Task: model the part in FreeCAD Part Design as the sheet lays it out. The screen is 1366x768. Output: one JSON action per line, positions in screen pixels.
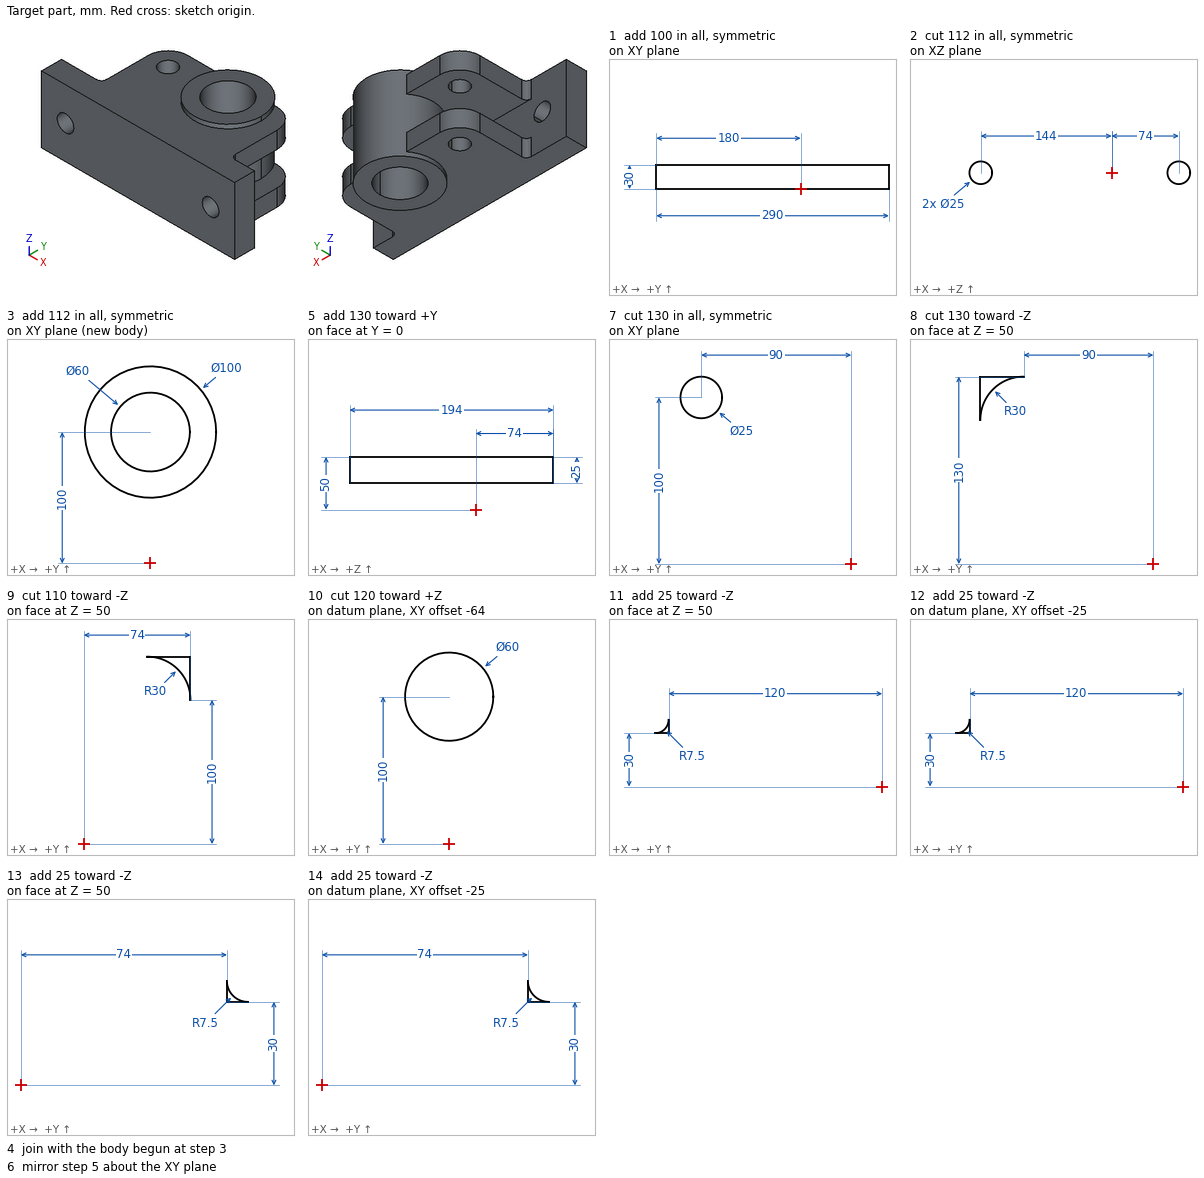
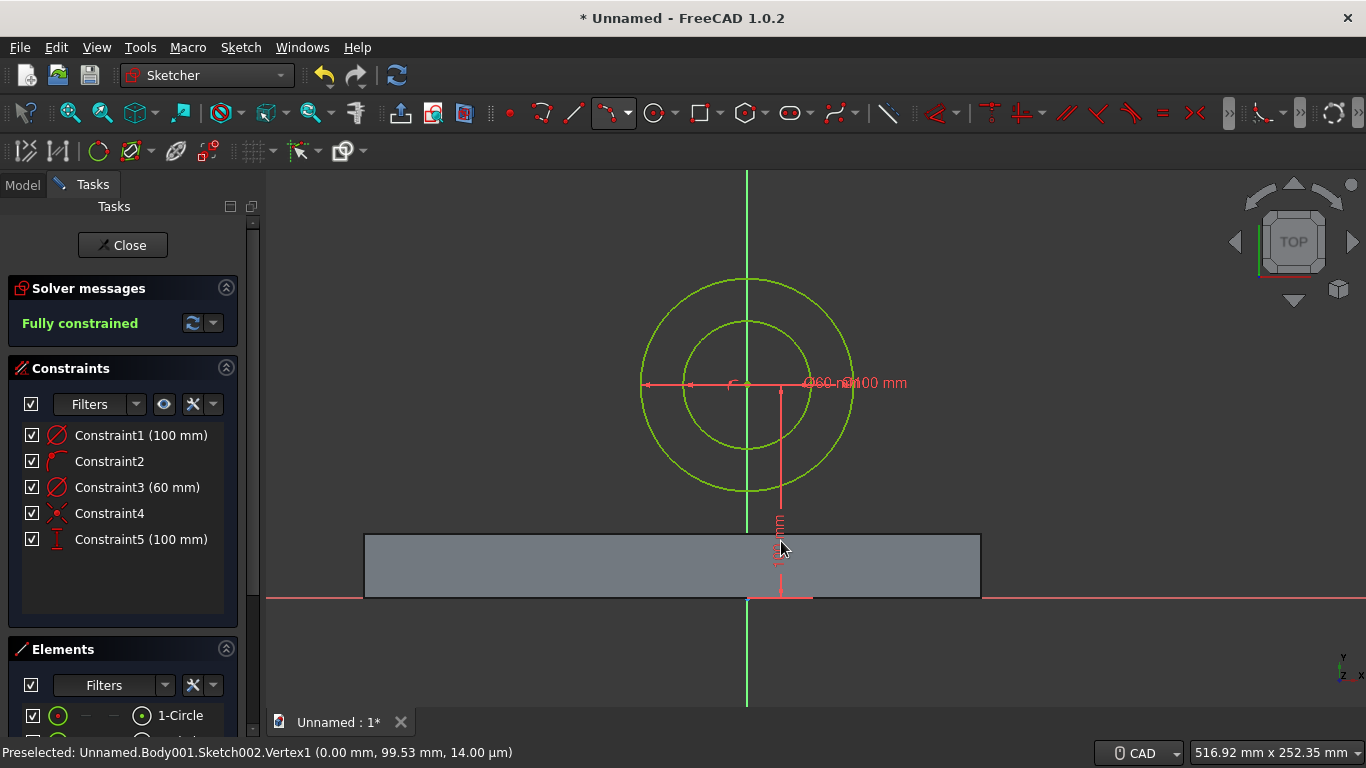
{"action": "left_click", "coordinate": [123, 245]}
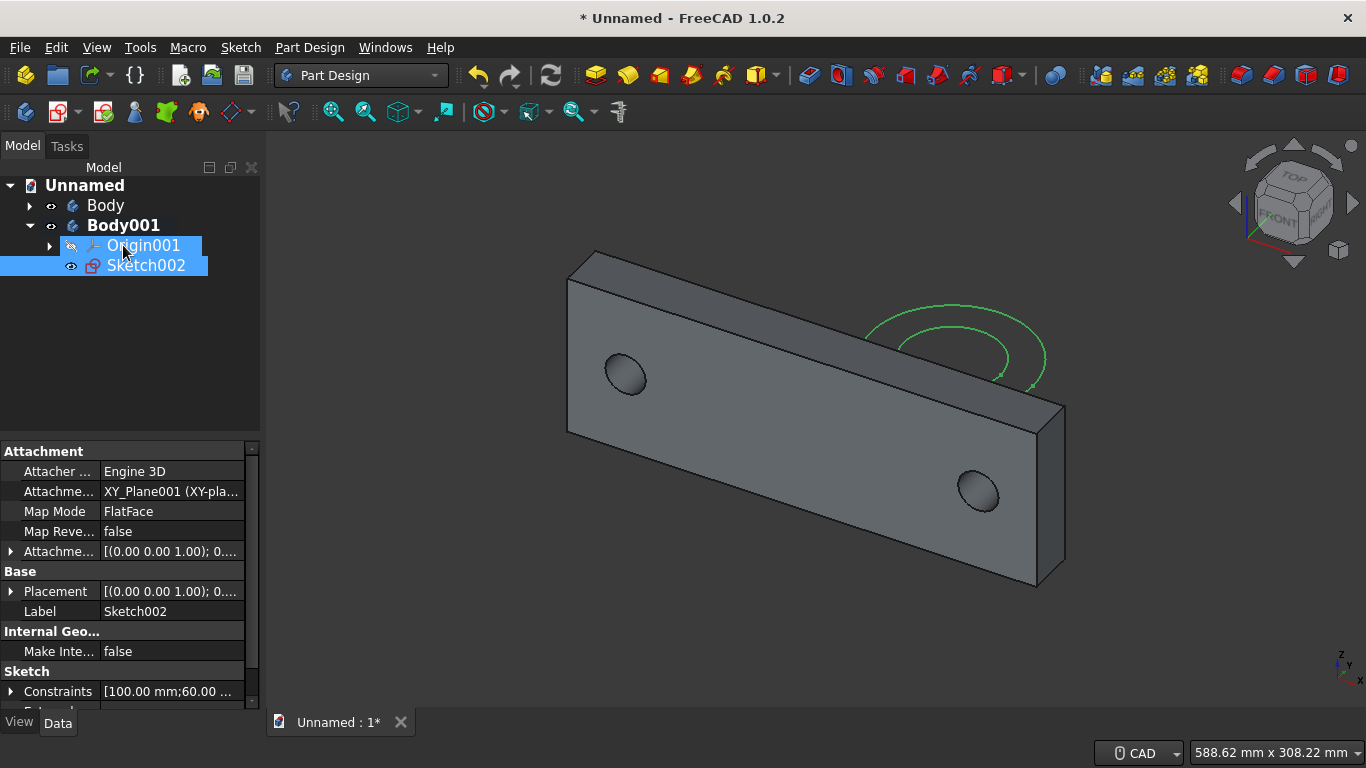
{"action": "left_click", "coordinate": [596, 76]}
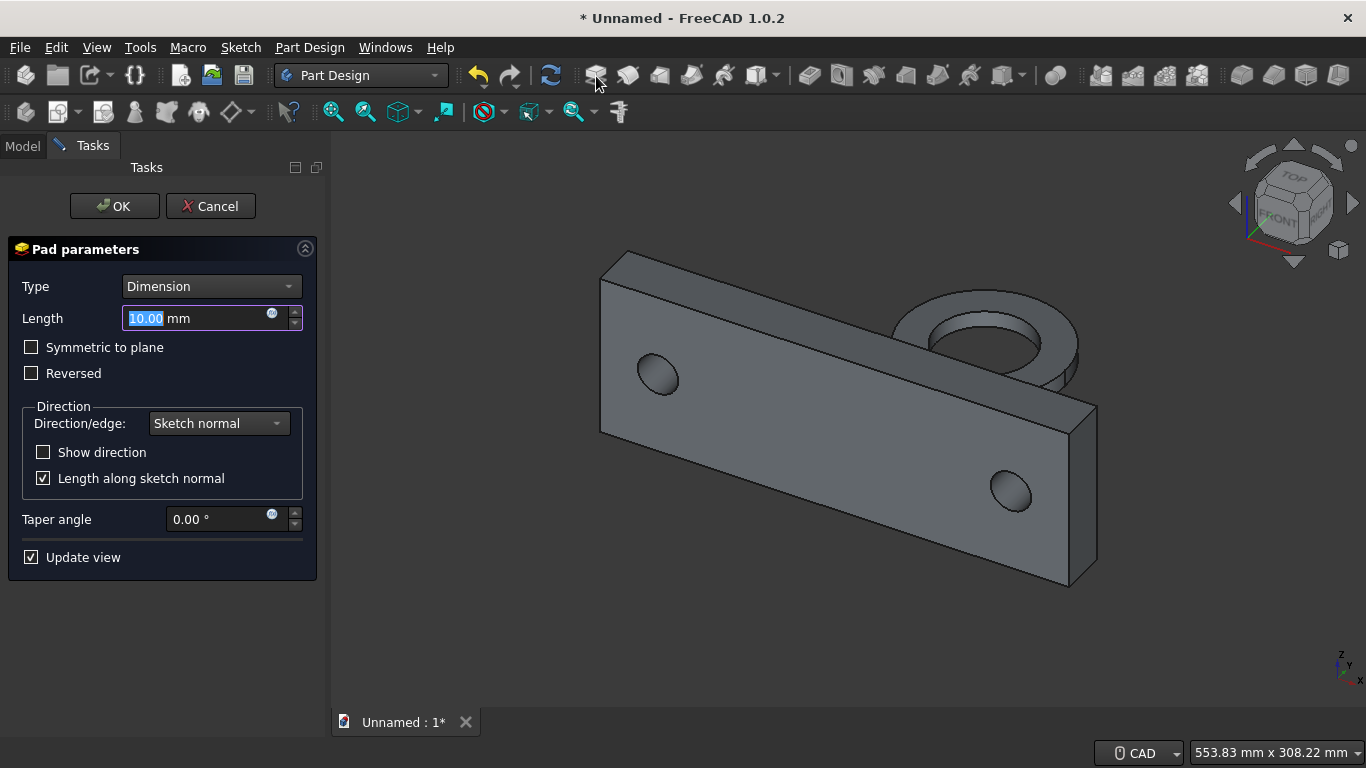
{"action": "type", "text": "112"}
{"action": "key", "text": "Tab"}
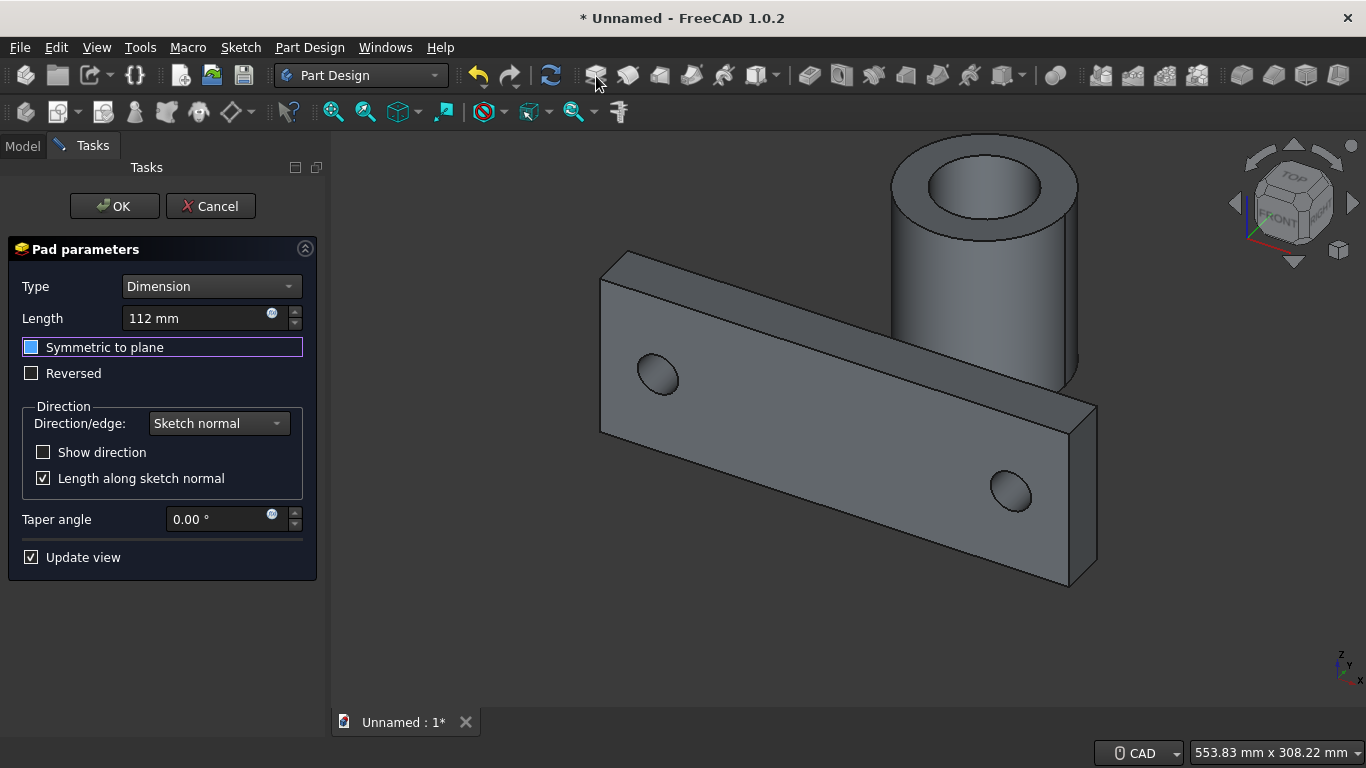
{"action": "left_click", "coordinate": [30, 347]}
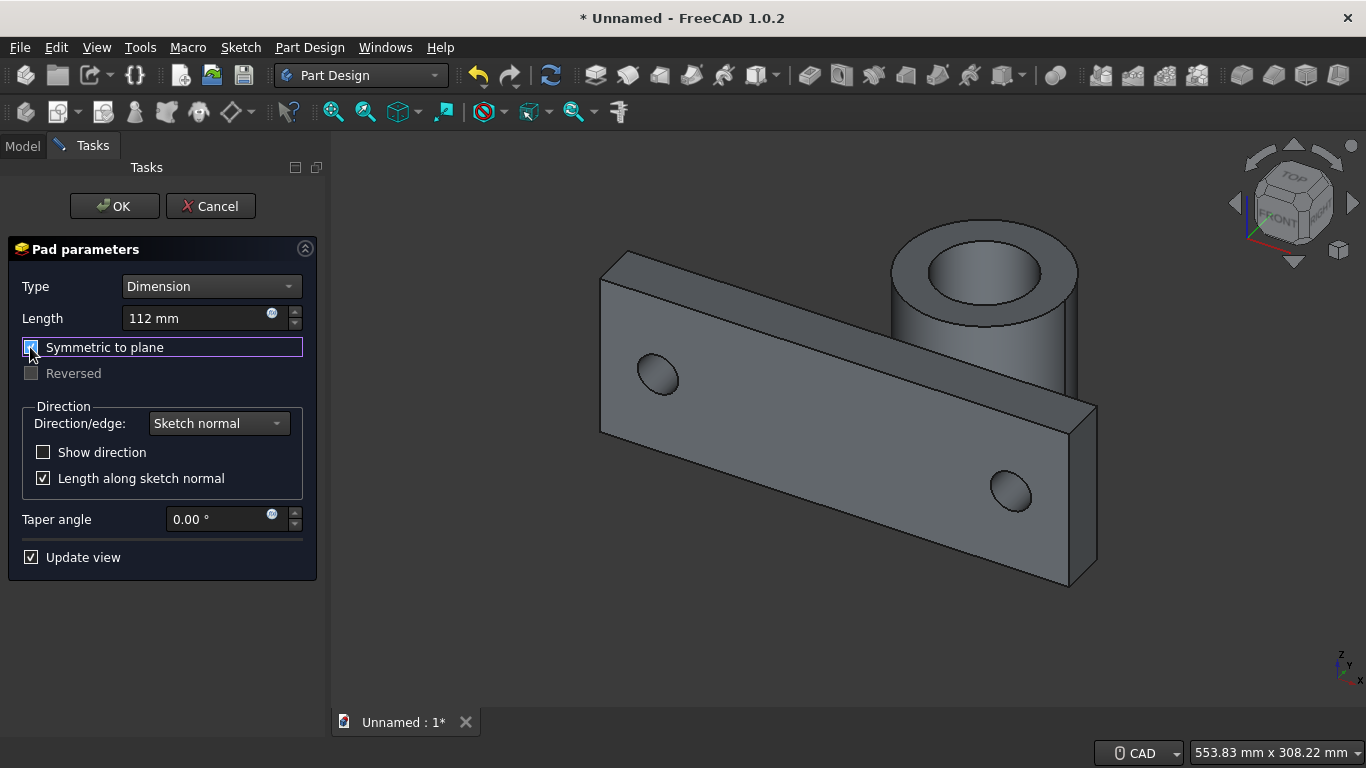
{"action": "left_click", "coordinate": [115, 206]}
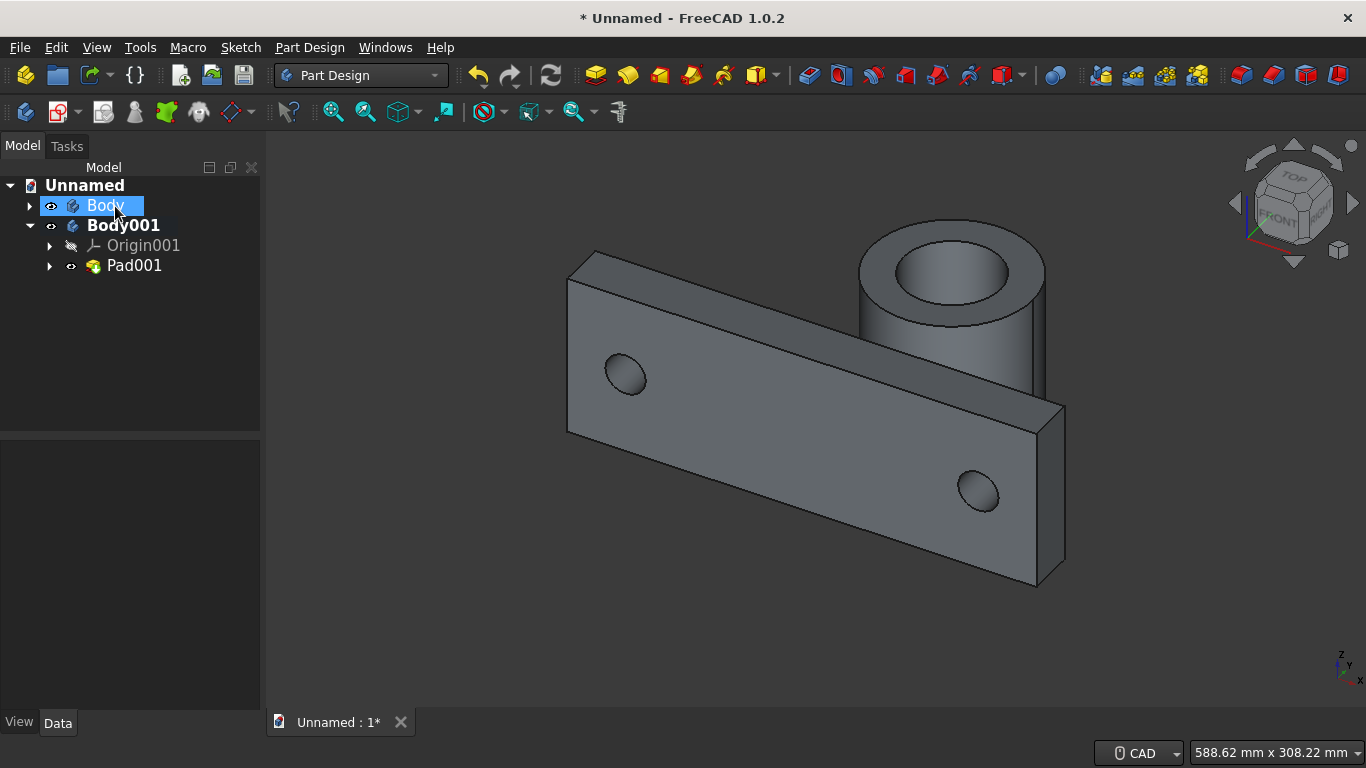
{"action": "double_click", "coordinate": [96, 206]}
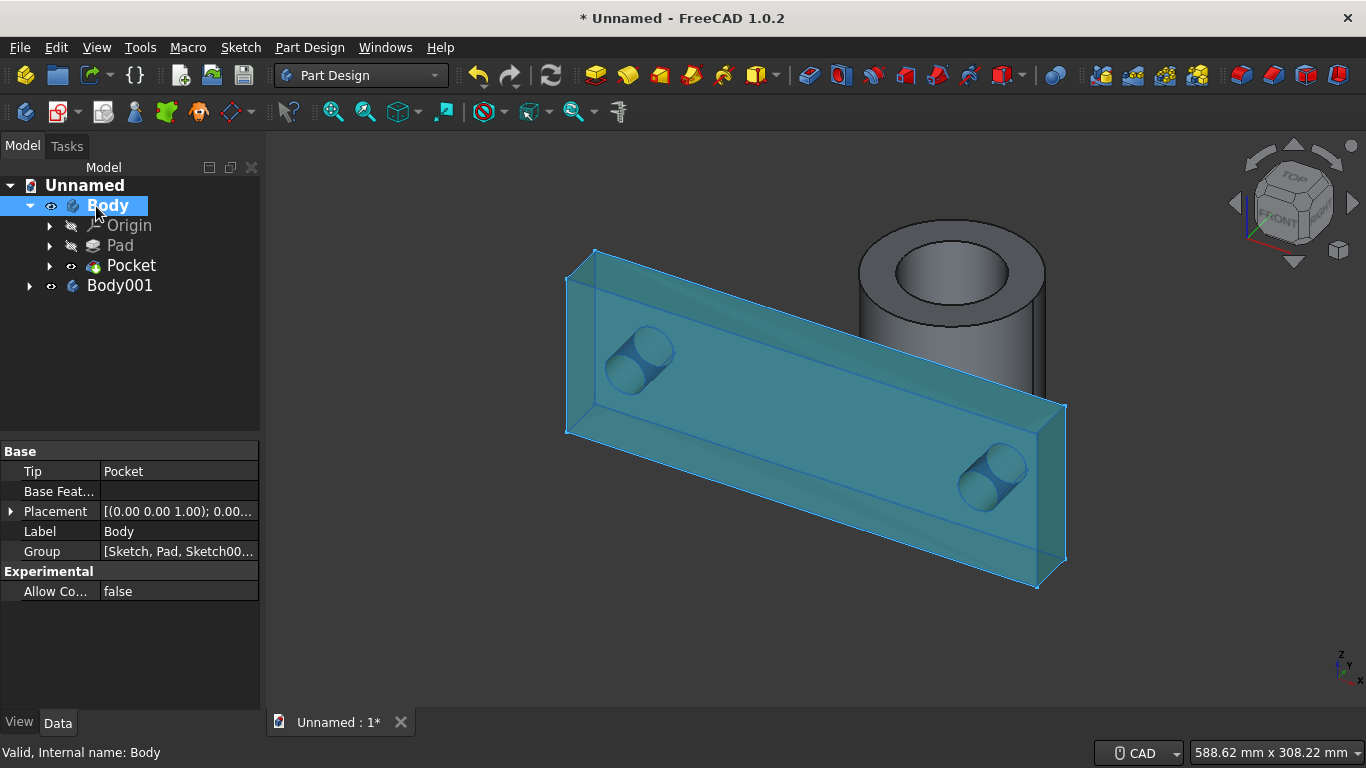
{"action": "left_click", "coordinate": [96, 206]}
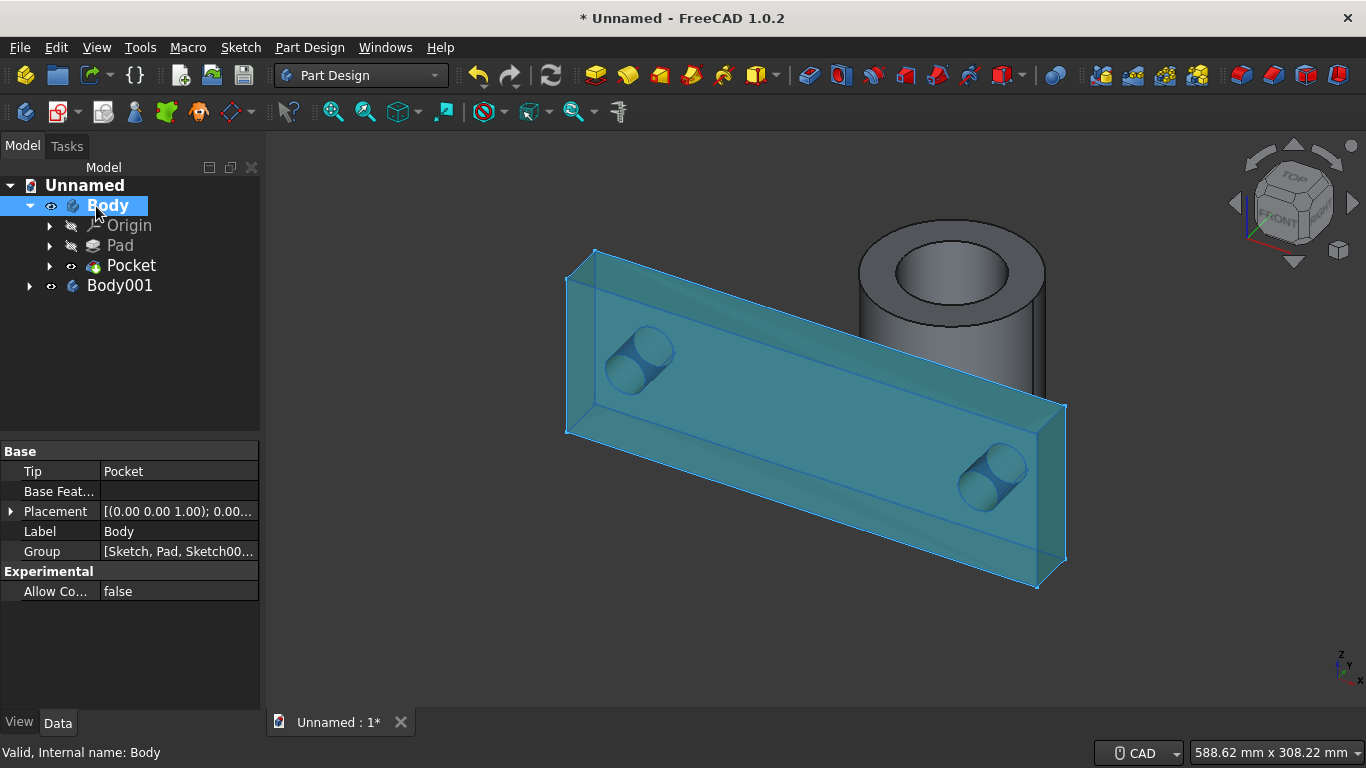
{"action": "left_click", "coordinate": [146, 591]}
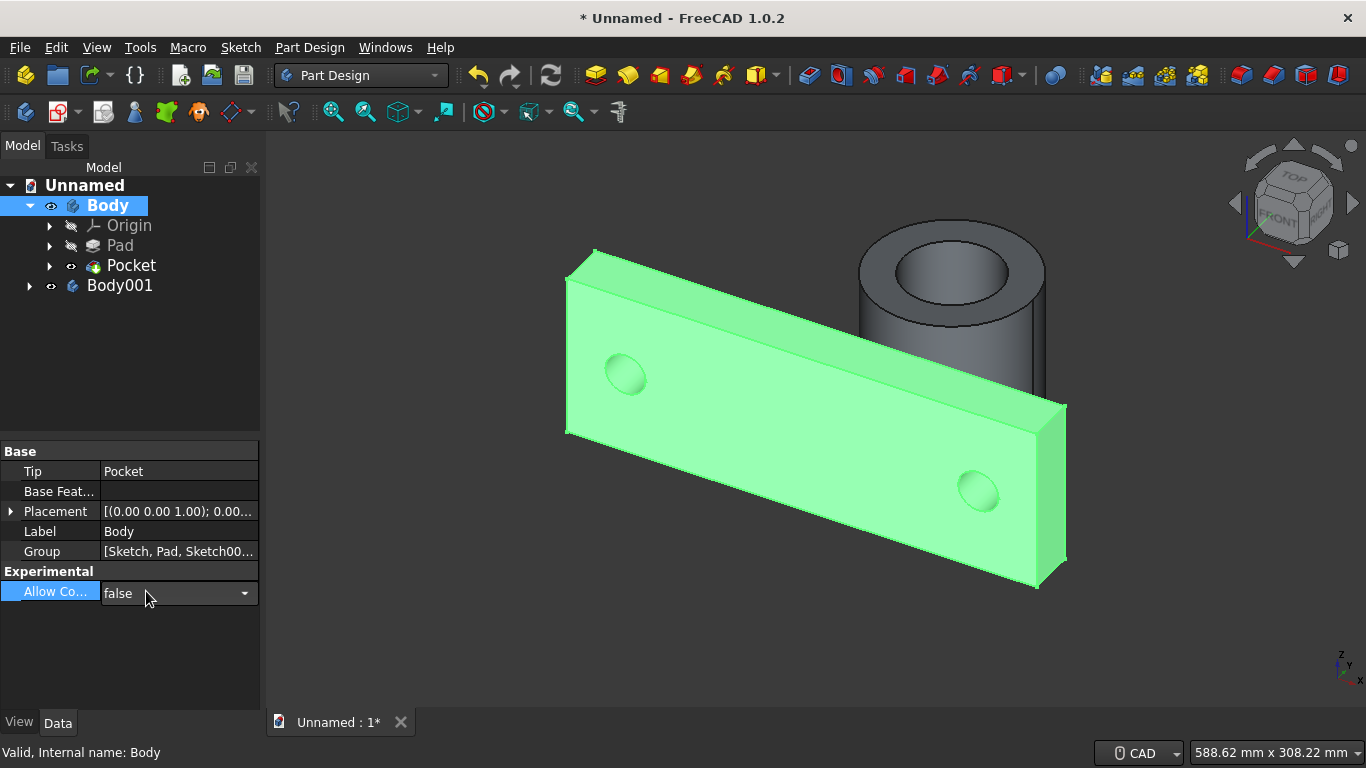
{"action": "left_click", "coordinate": [146, 591]}